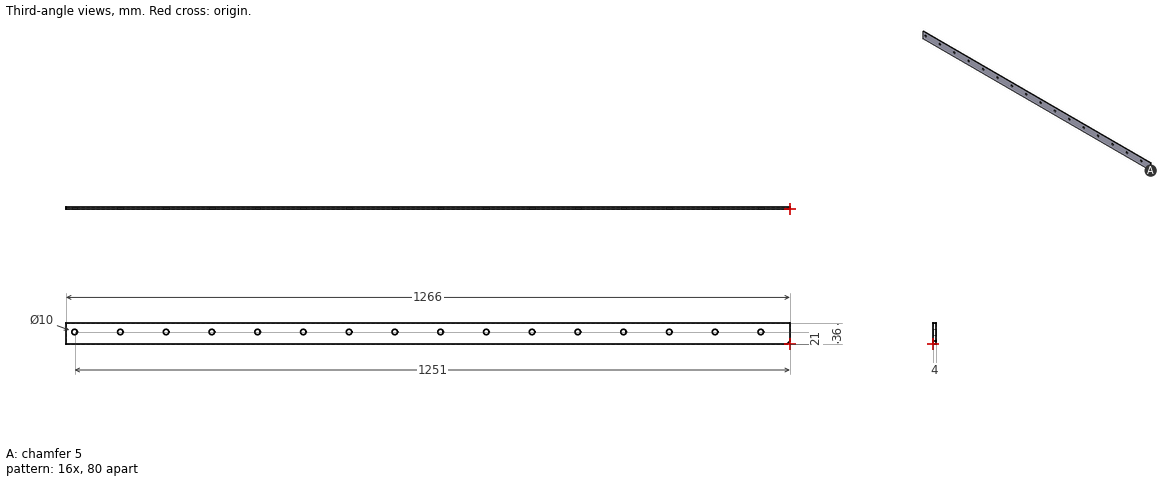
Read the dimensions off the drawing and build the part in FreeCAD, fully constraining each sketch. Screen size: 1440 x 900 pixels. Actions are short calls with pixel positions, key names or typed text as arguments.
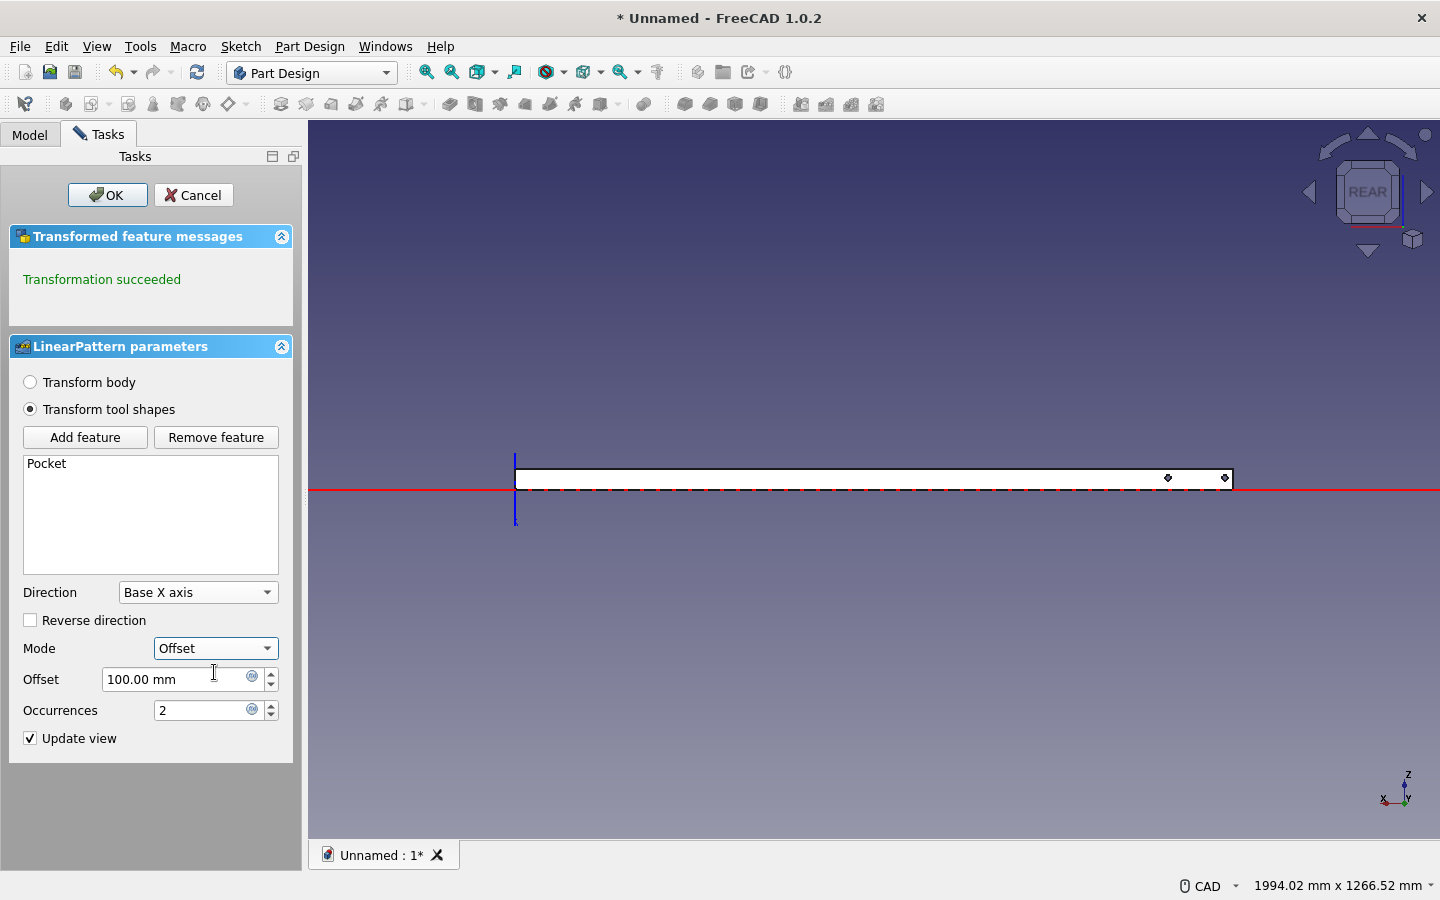
triple_click(184, 680)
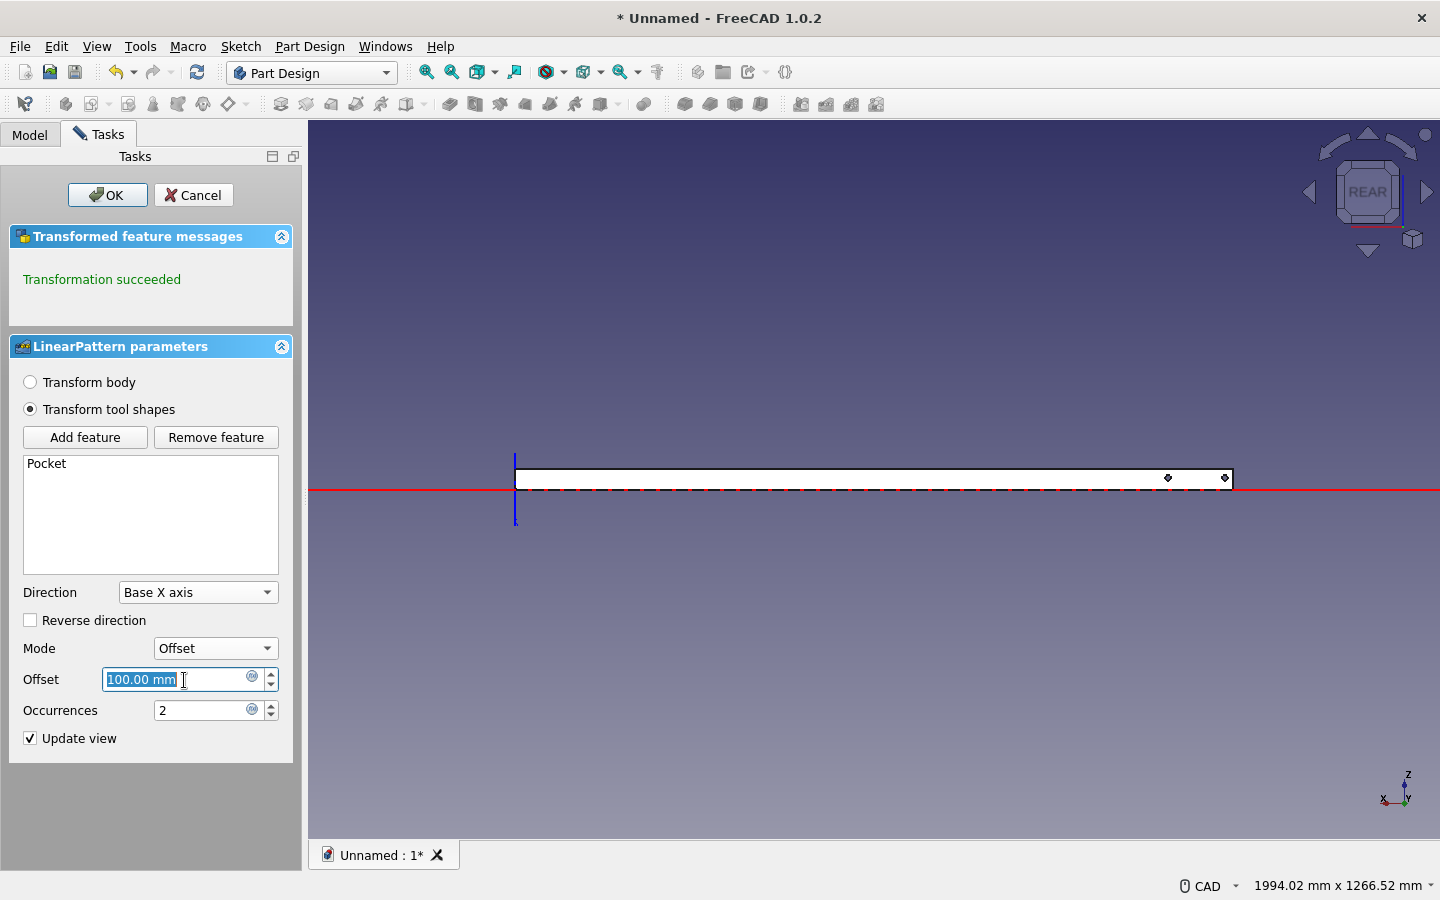
text(80)
key(Tab)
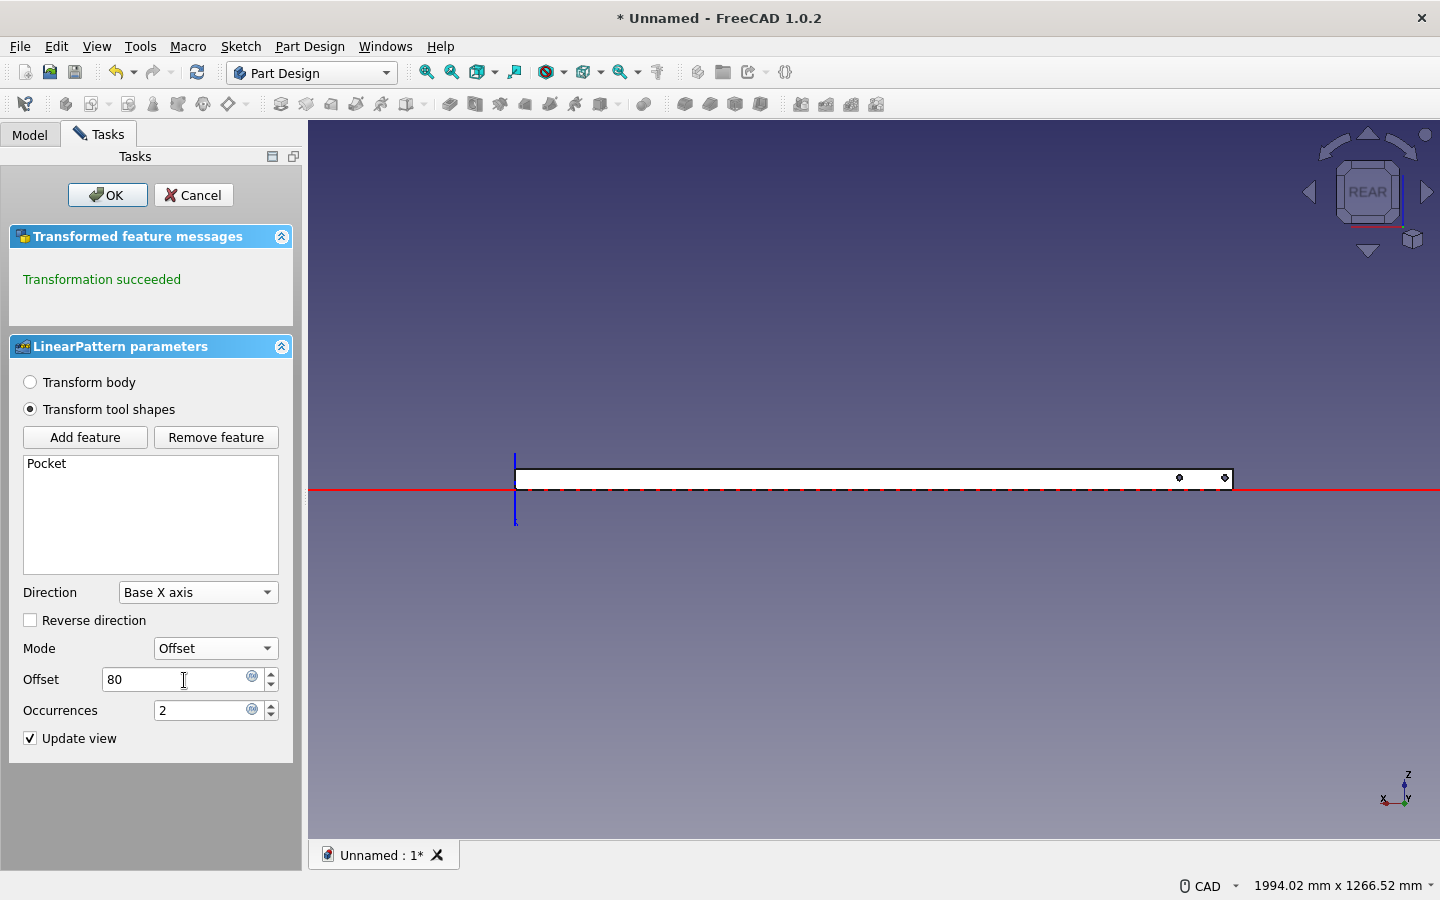
triple_click(210, 710)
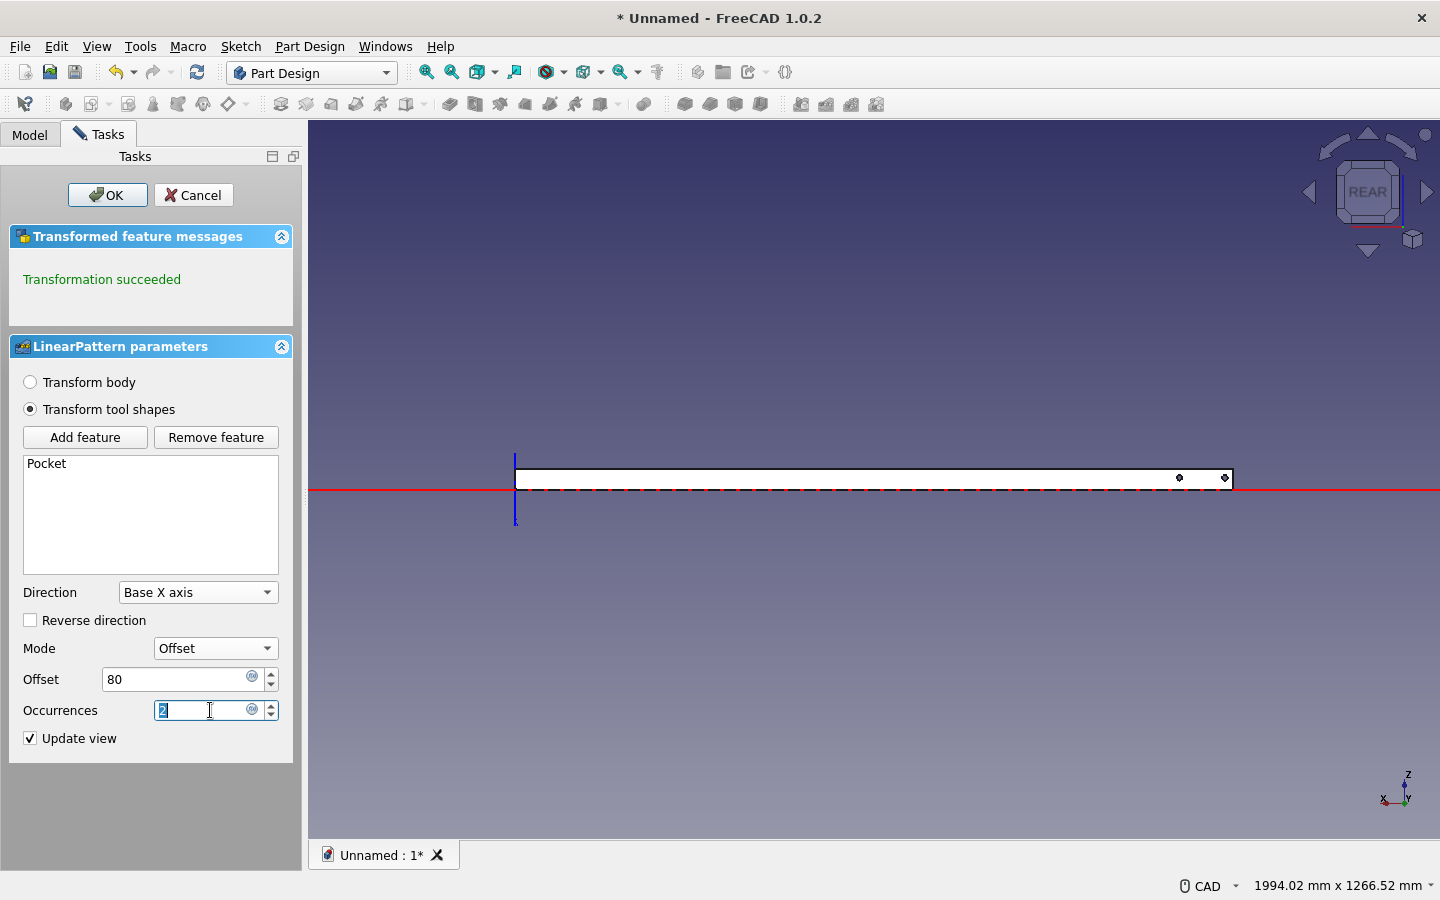
text(16)
key(Tab)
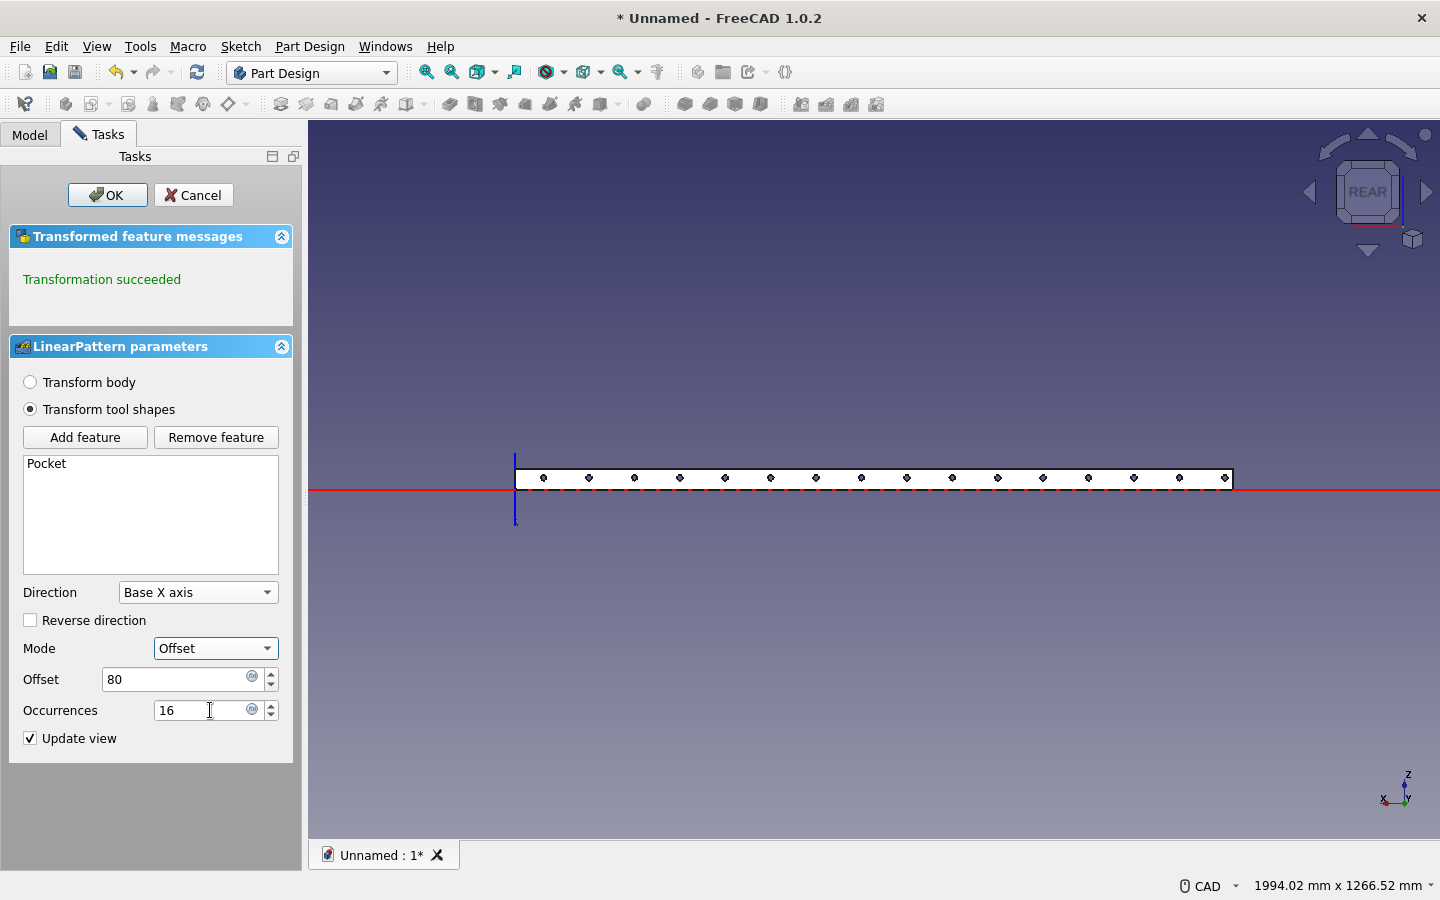
click(108, 195)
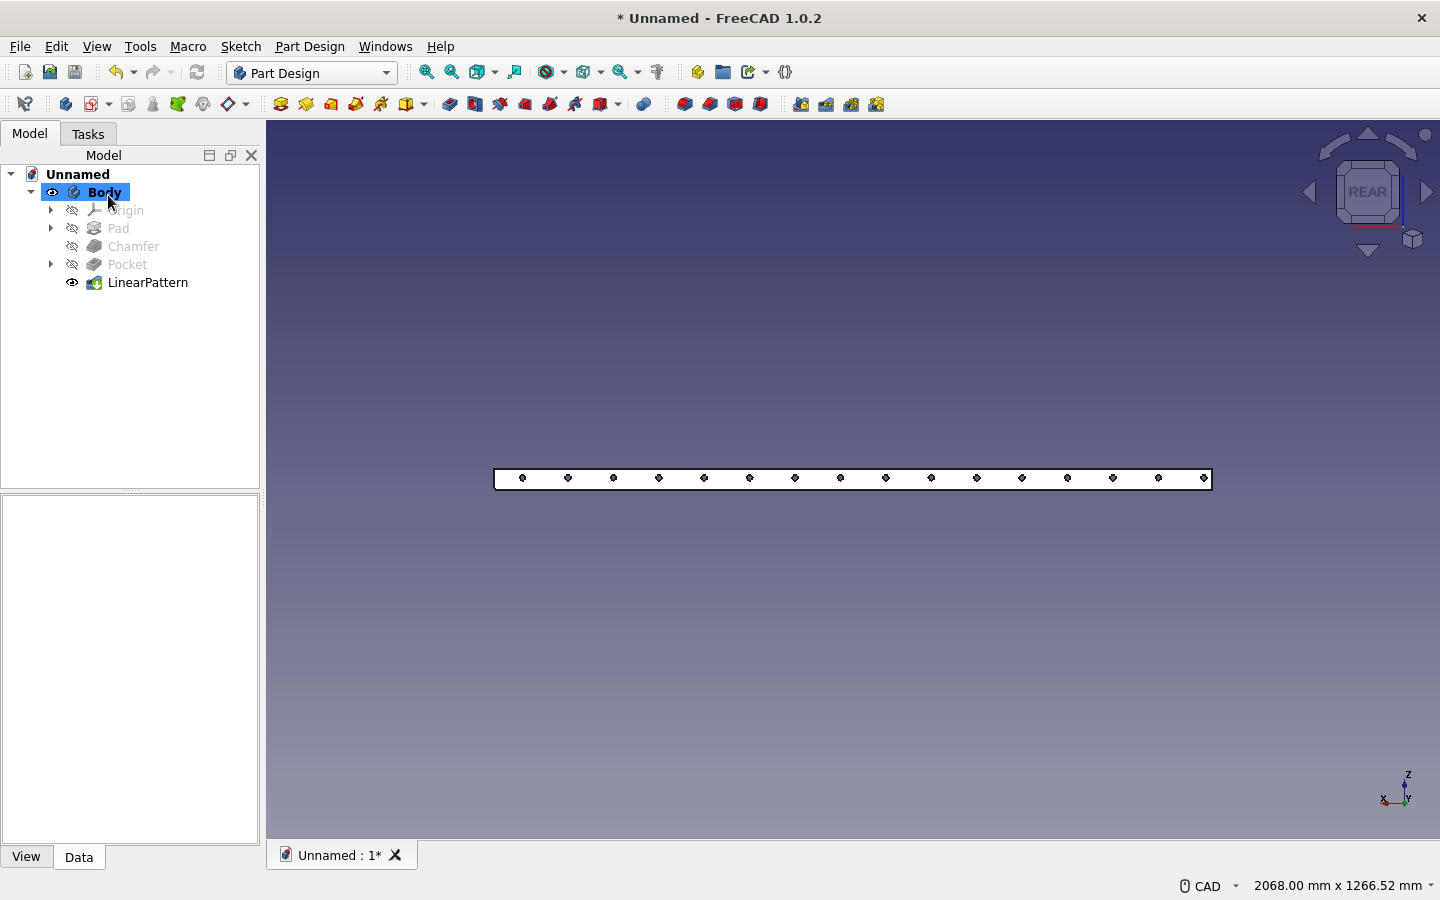
key(0)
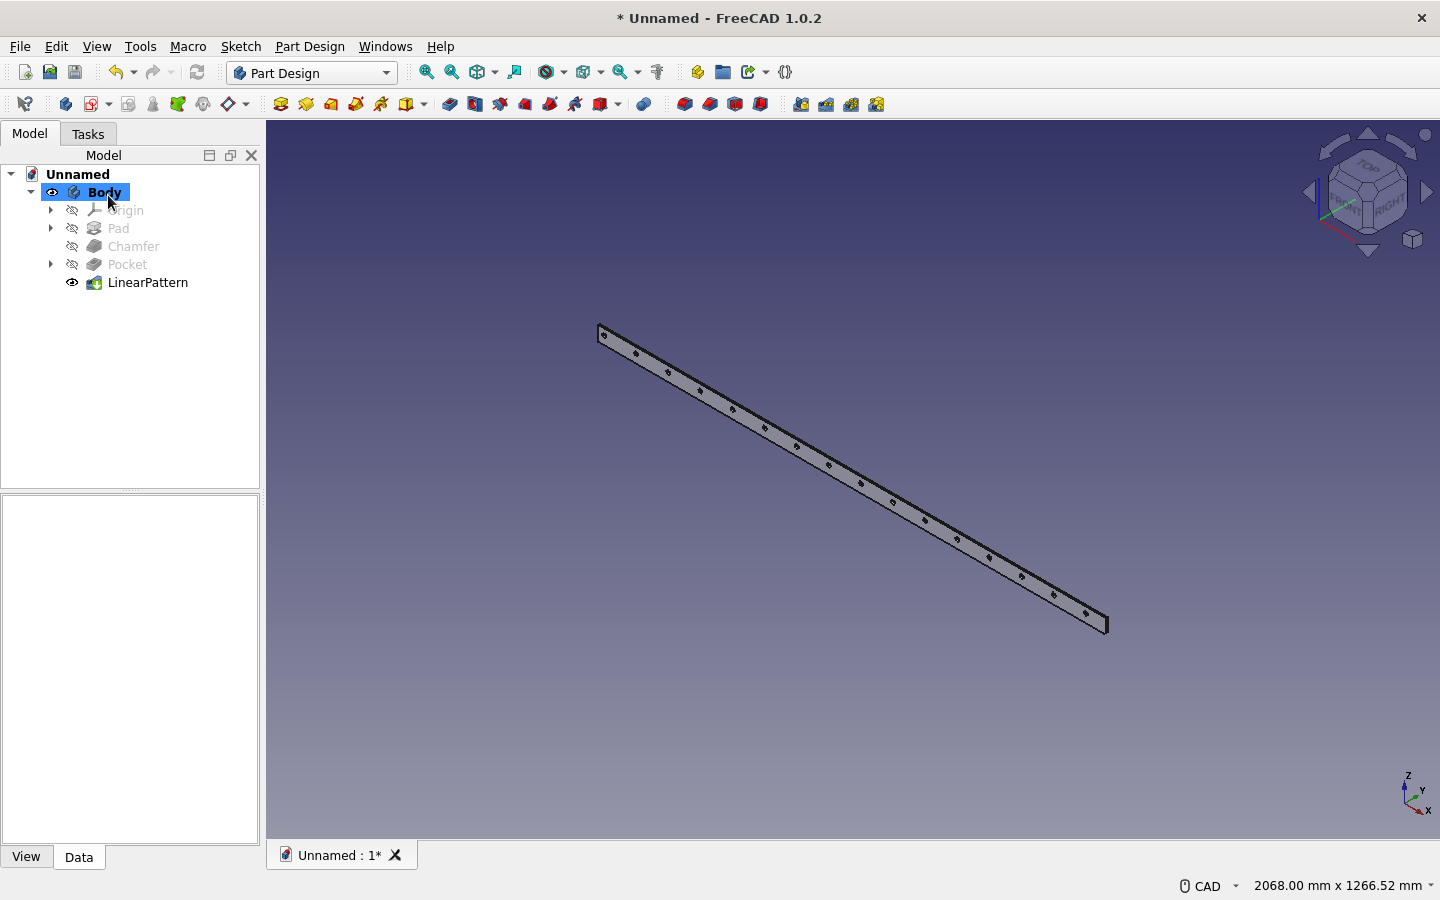
click(427, 72)